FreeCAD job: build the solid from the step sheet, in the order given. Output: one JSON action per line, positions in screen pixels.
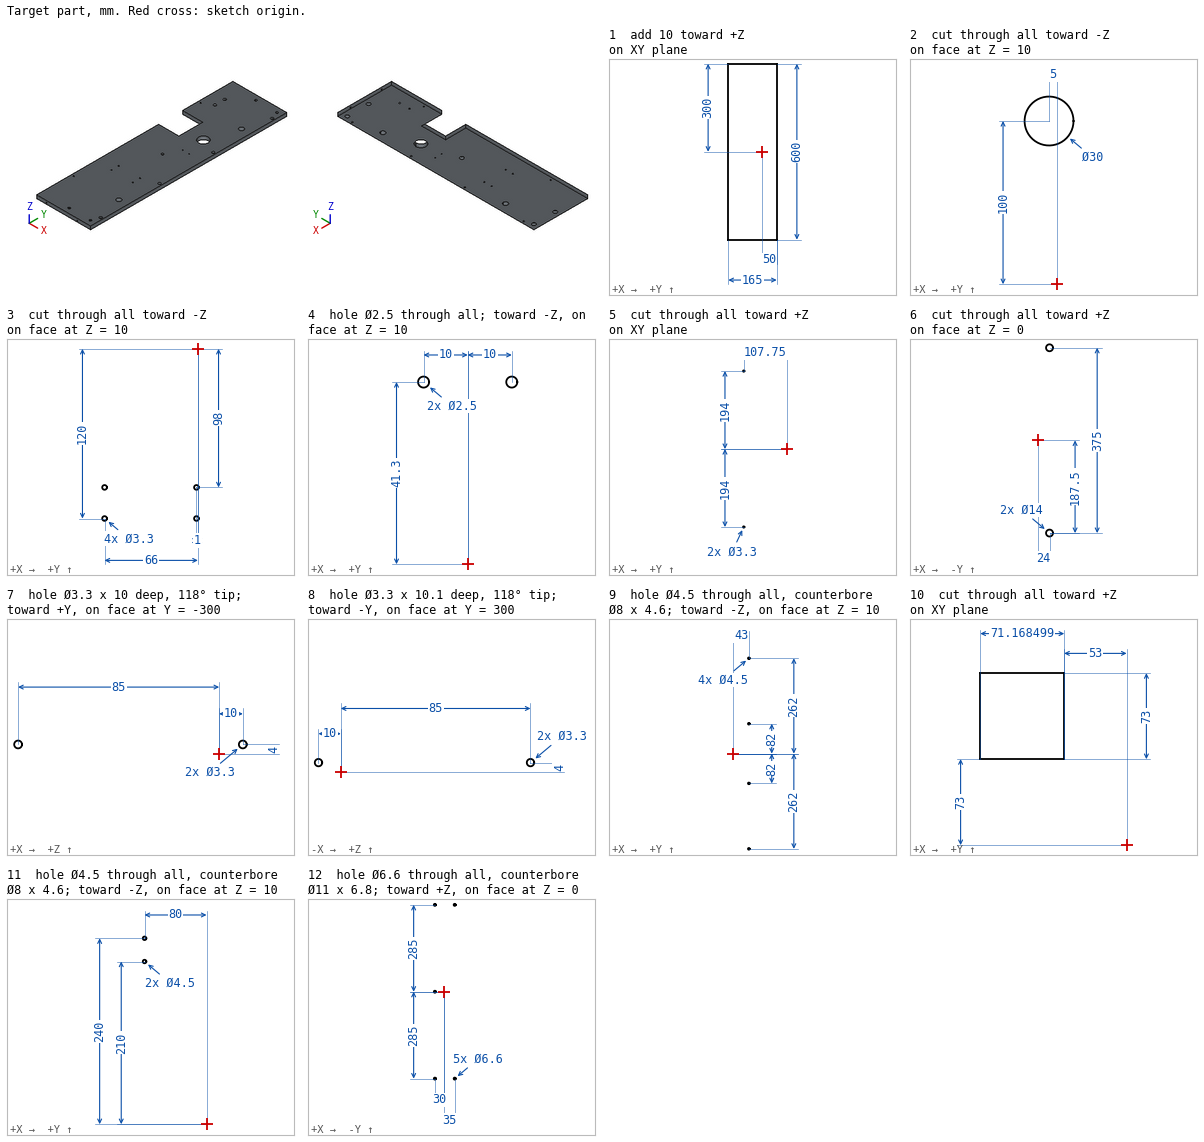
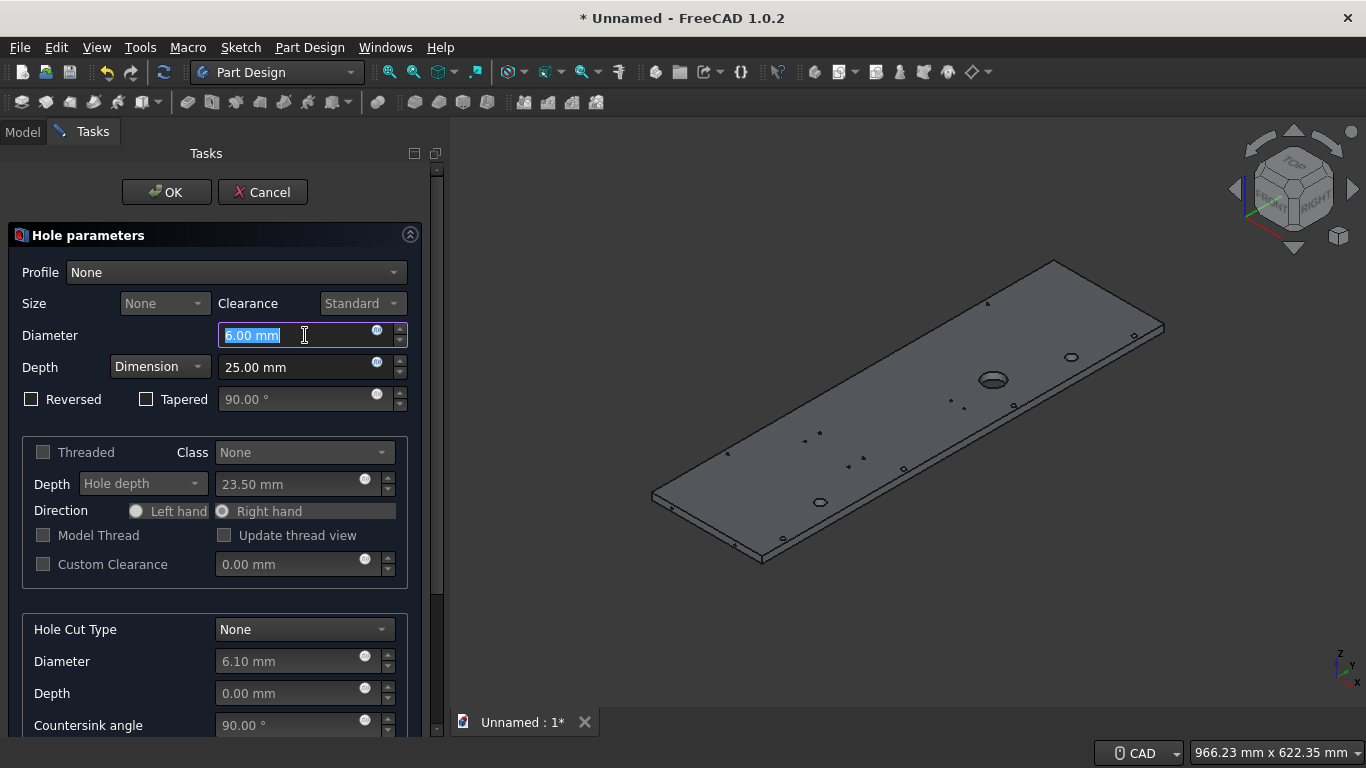
{"action": "type", "text": "4.5"}
{"action": "key", "text": "Tab"}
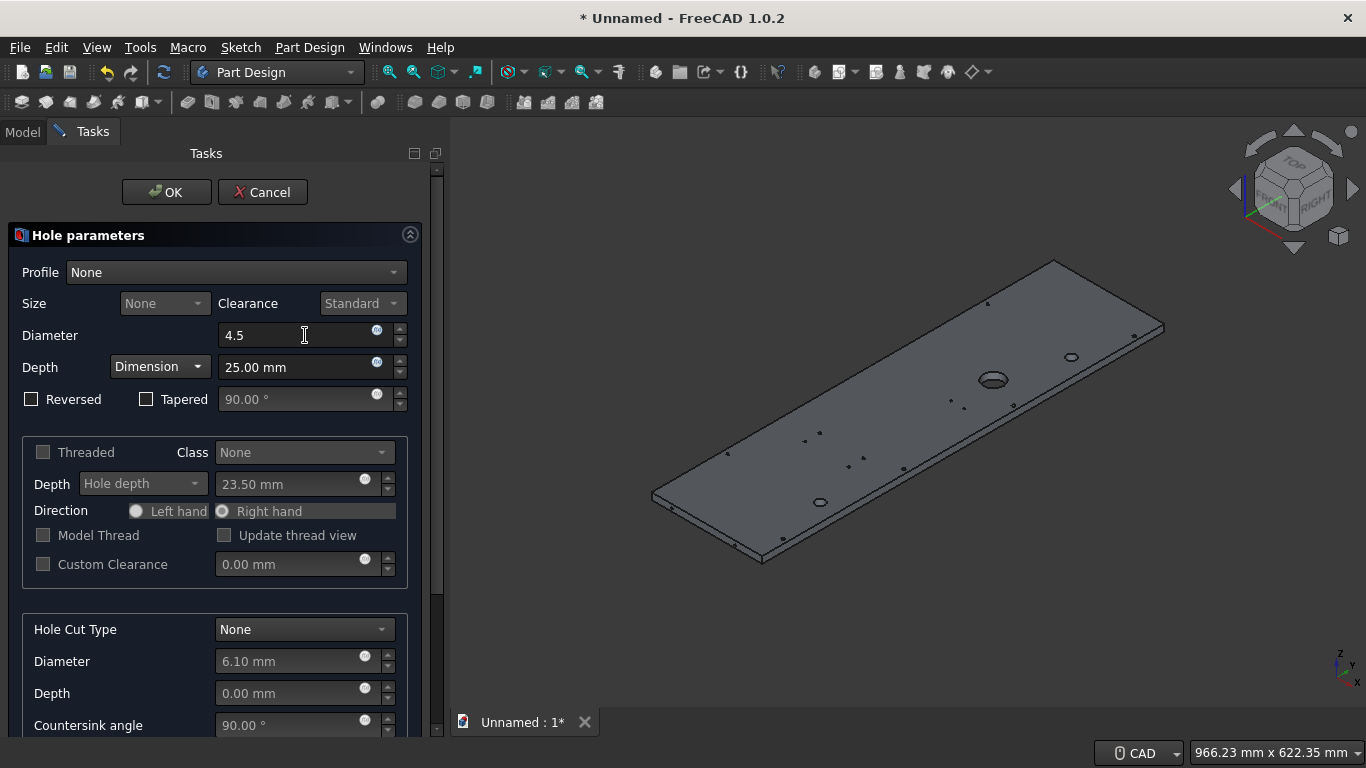
{"action": "left_click", "coordinate": [161, 366]}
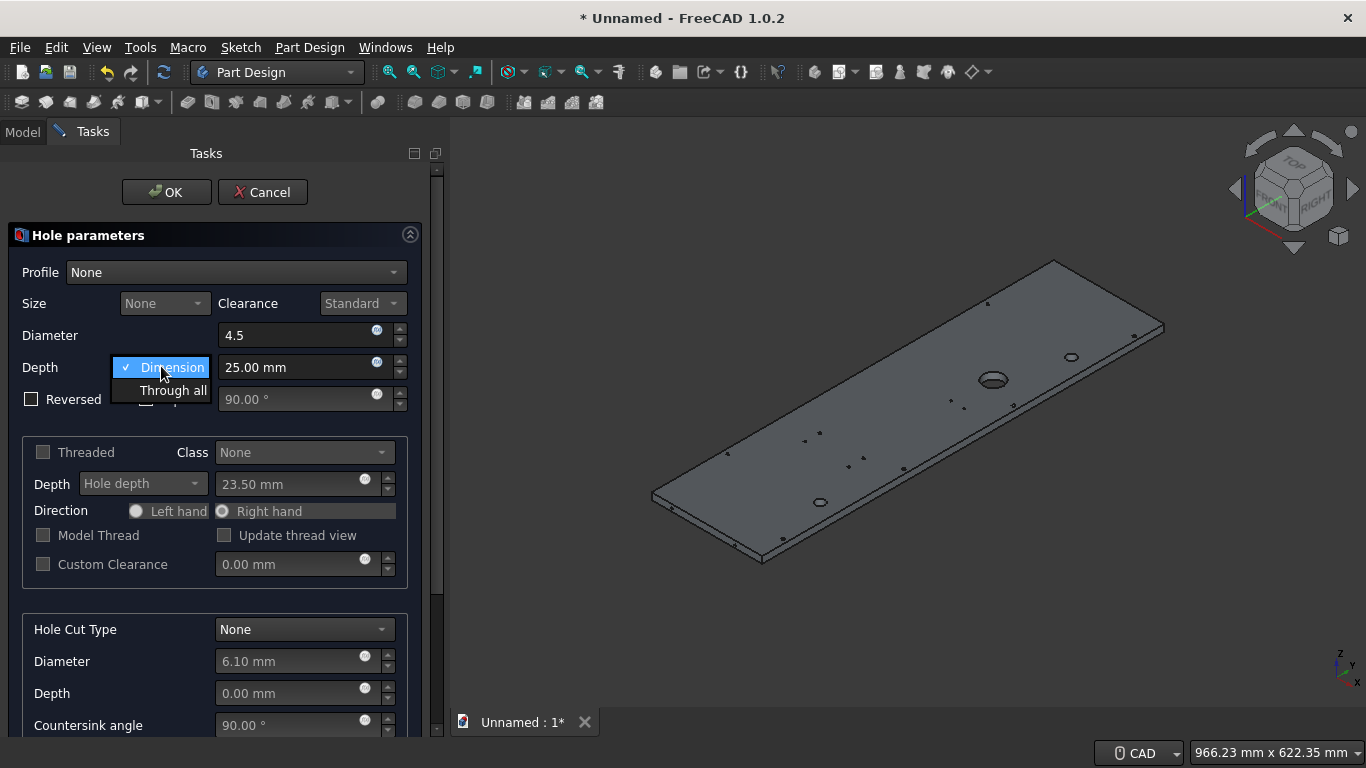
{"action": "left_click", "coordinate": [160, 390]}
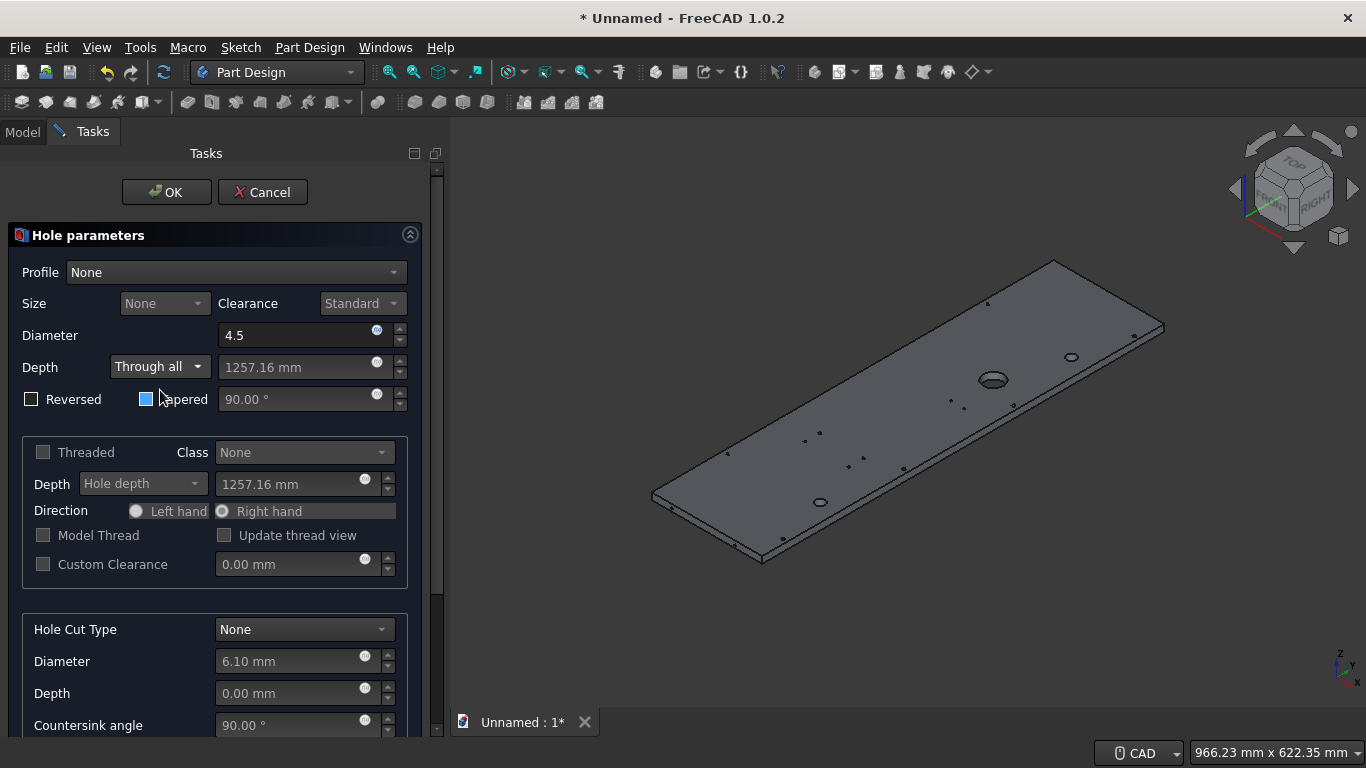
{"action": "left_click", "coordinate": [306, 630]}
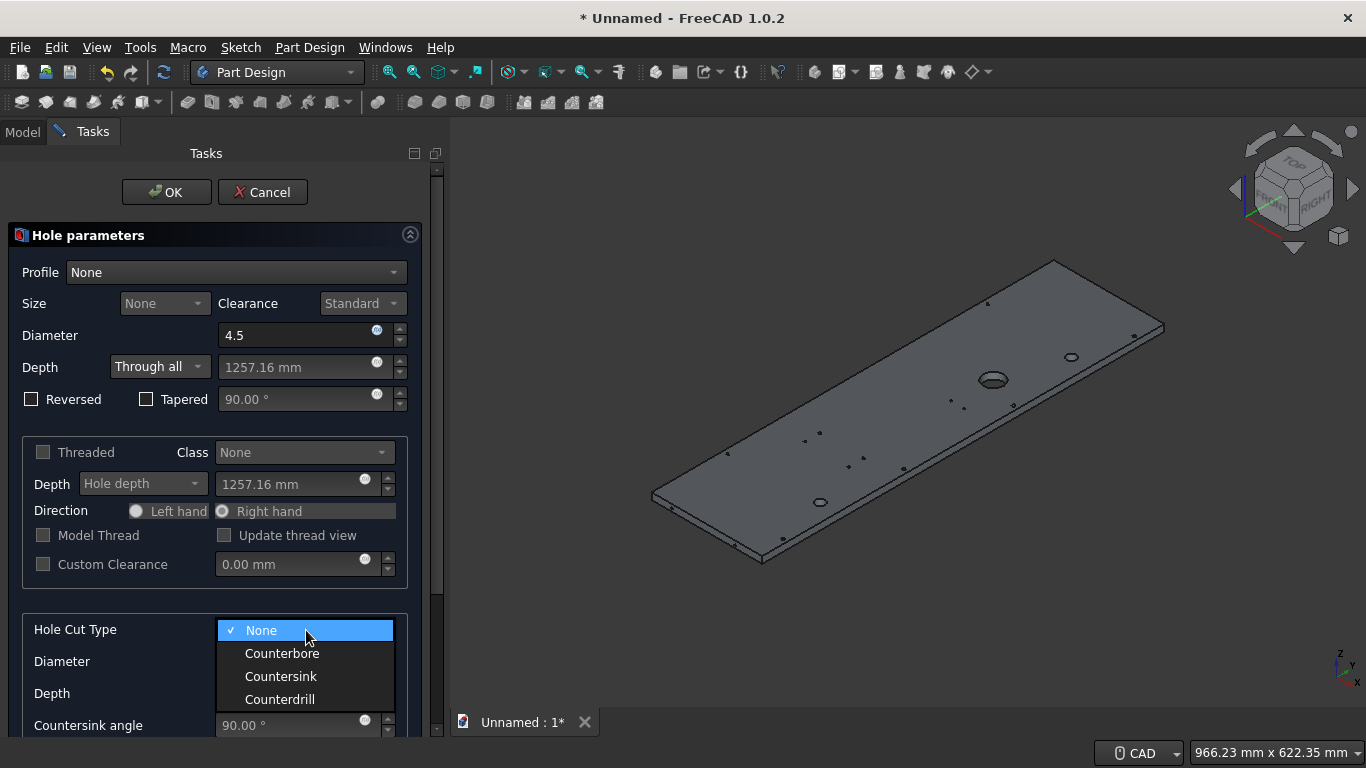
{"action": "left_click", "coordinate": [304, 654]}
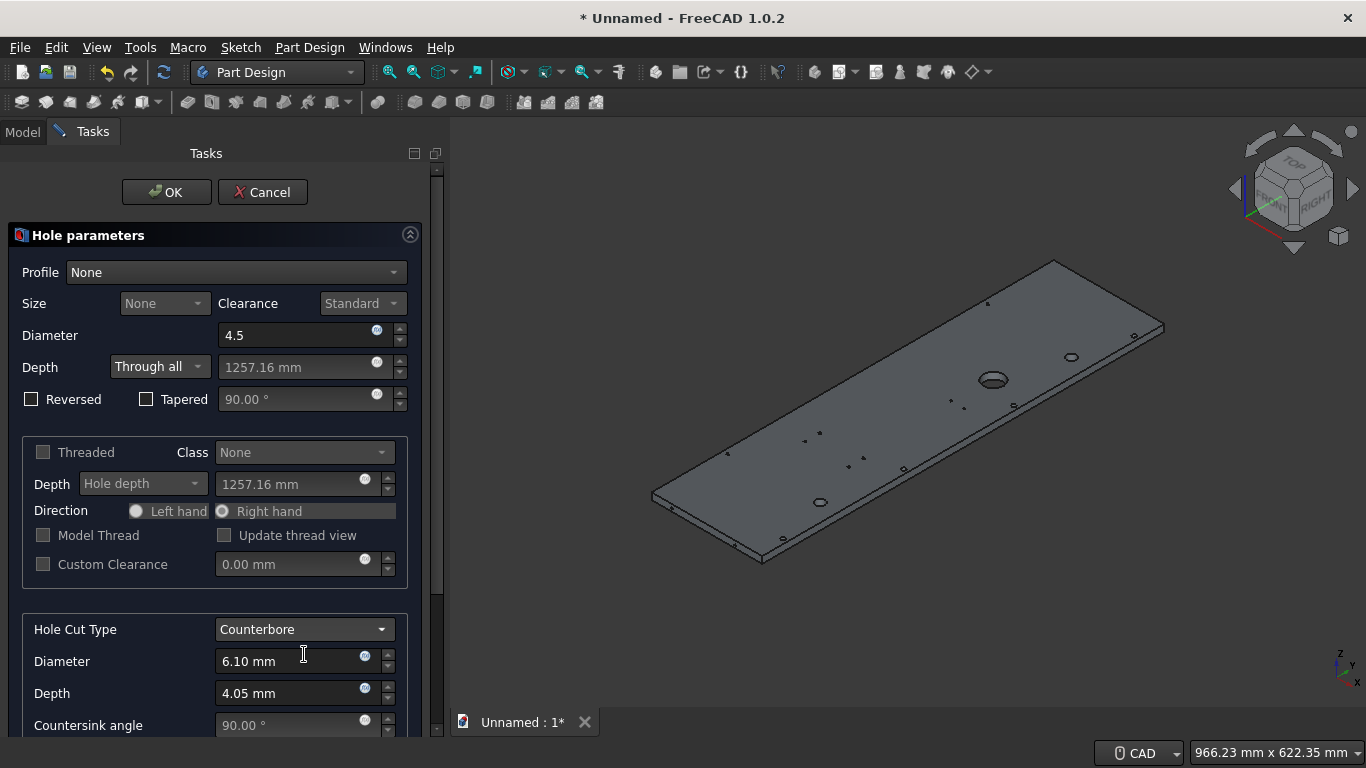
{"action": "triple_click", "coordinate": [298, 661]}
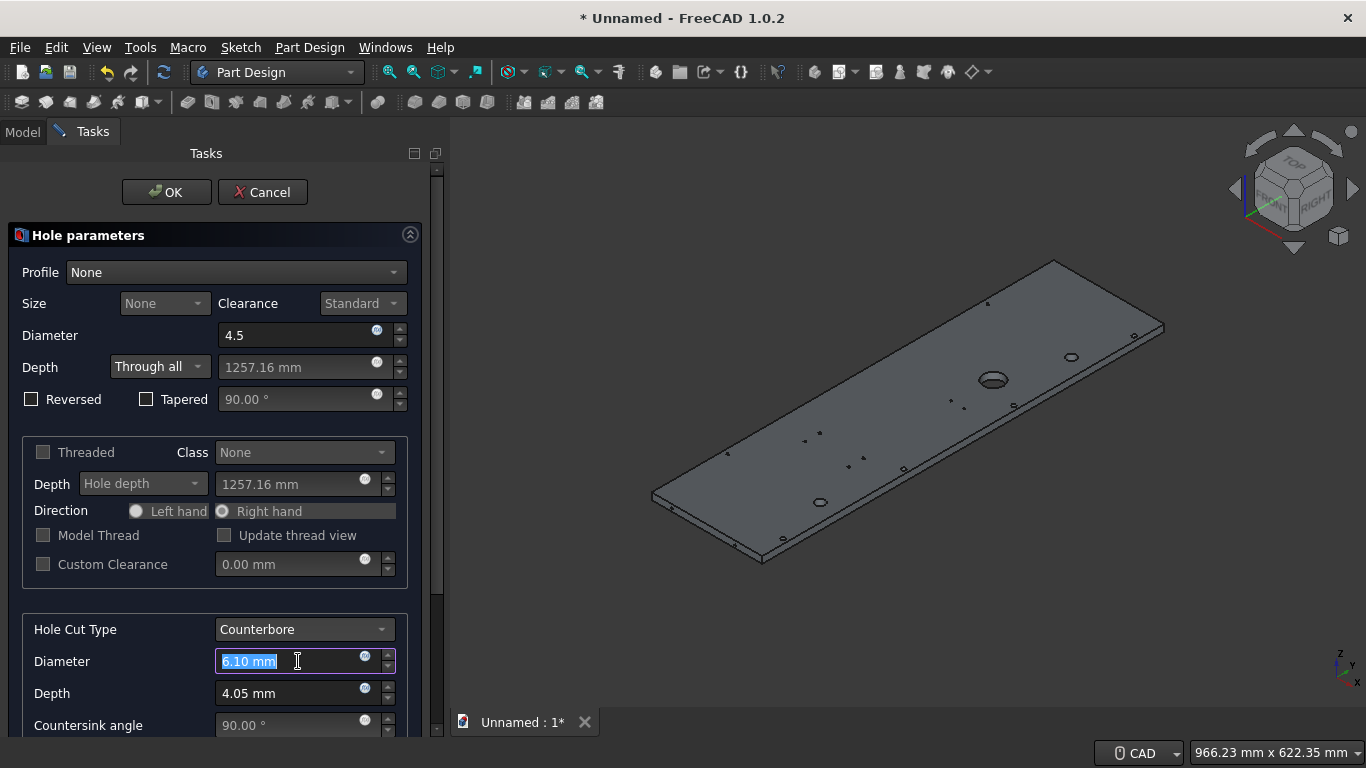
{"action": "type", "text": "8"}
{"action": "key", "text": "Tab"}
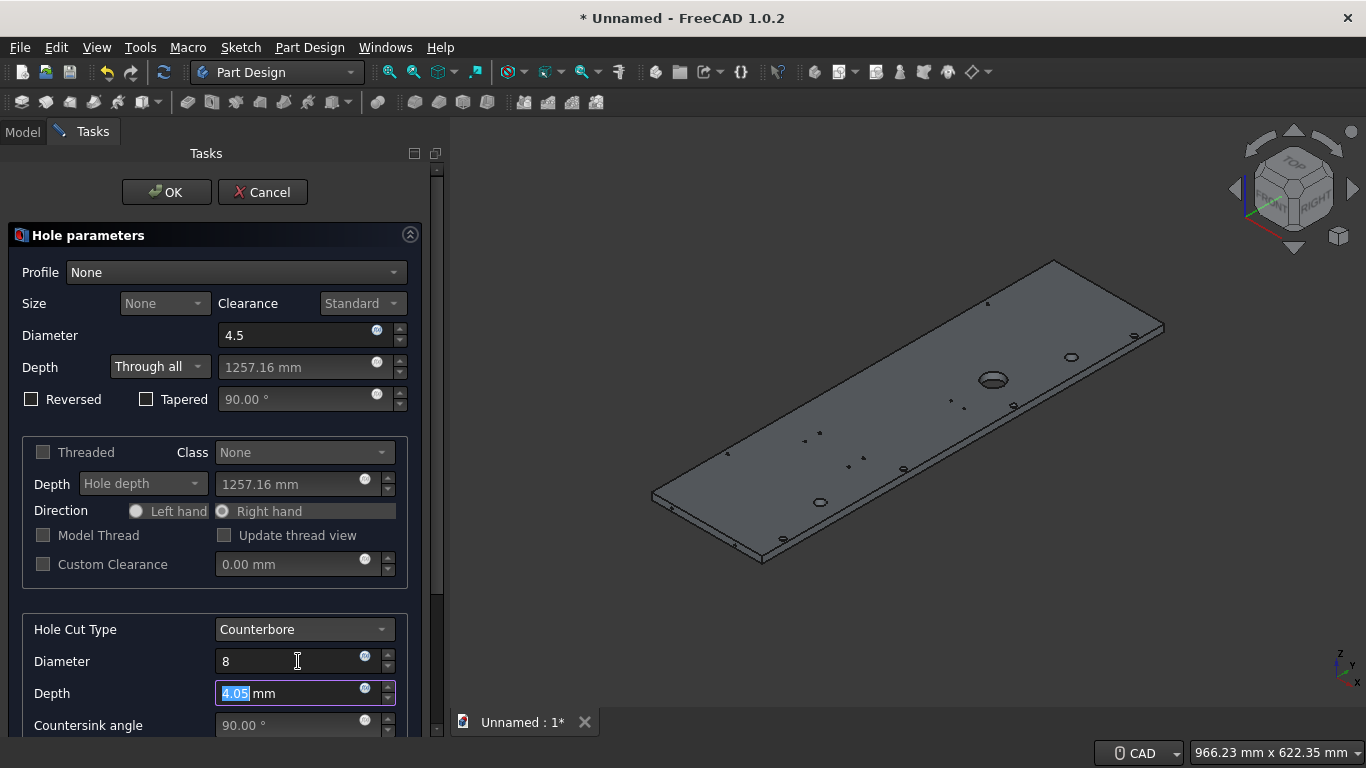
{"action": "type", "text": "4.6"}
{"action": "key", "text": "Tab"}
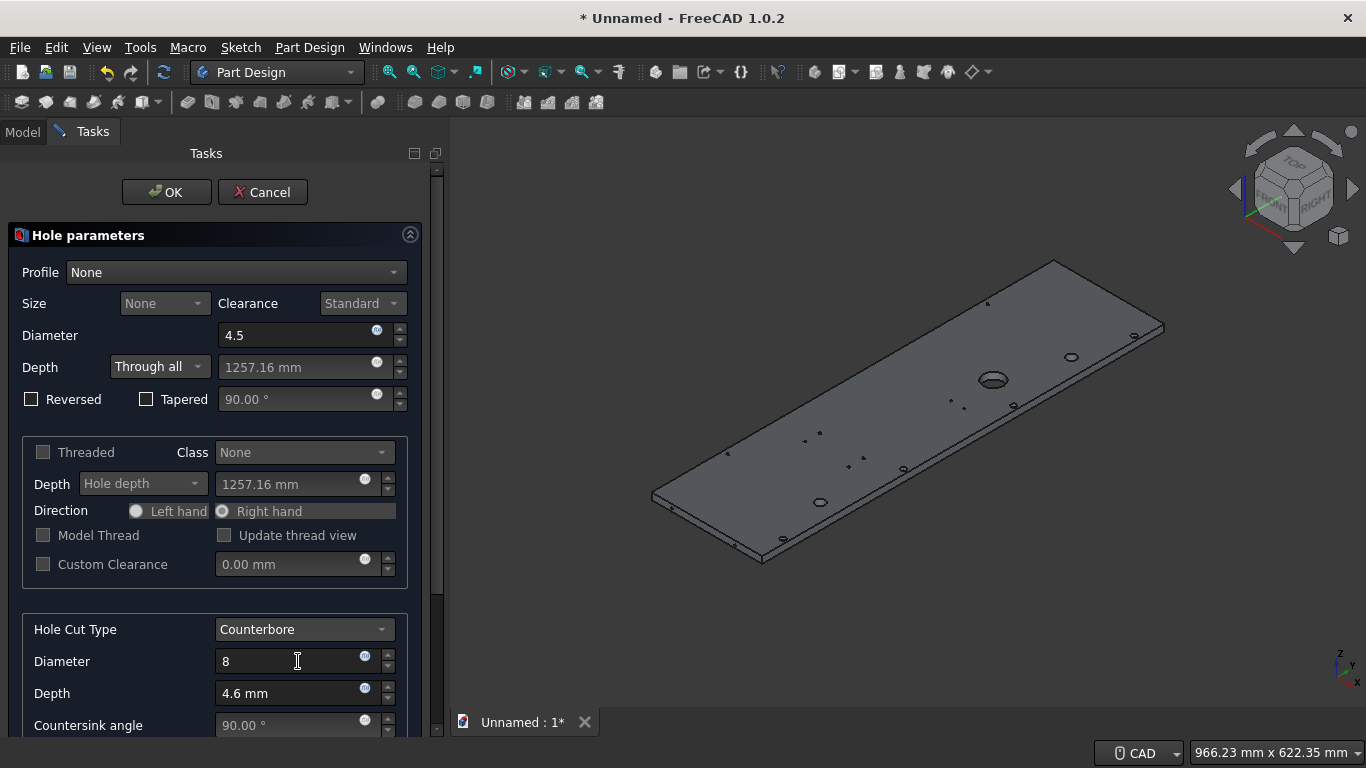
{"action": "left_click", "coordinate": [167, 192]}